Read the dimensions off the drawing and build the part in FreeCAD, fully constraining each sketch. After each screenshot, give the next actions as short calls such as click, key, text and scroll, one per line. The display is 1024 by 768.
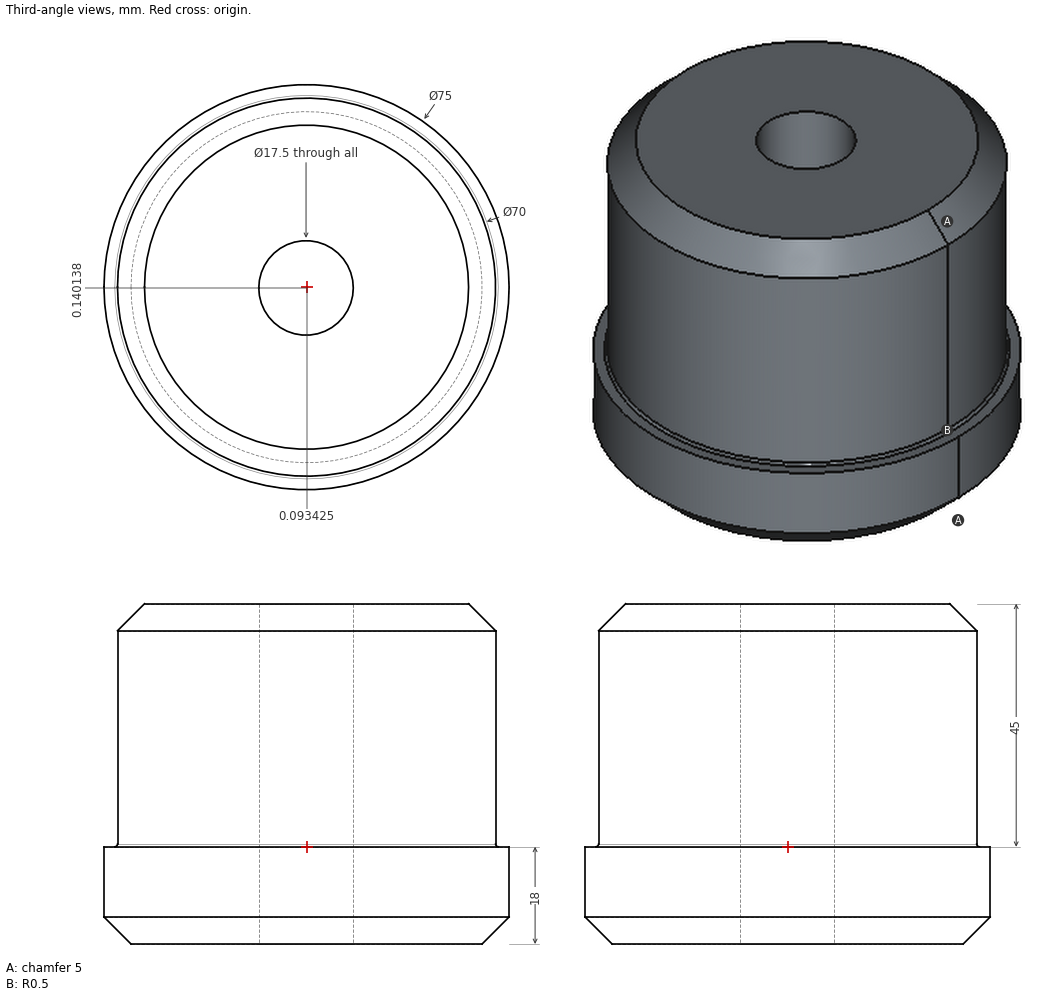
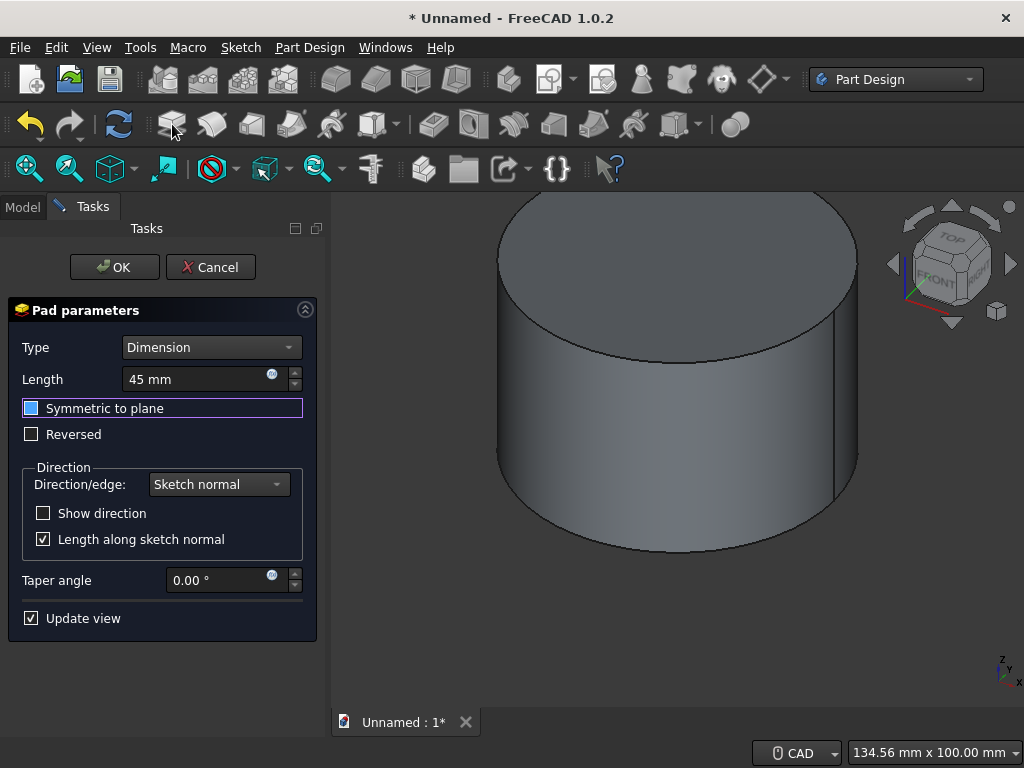
click(115, 267)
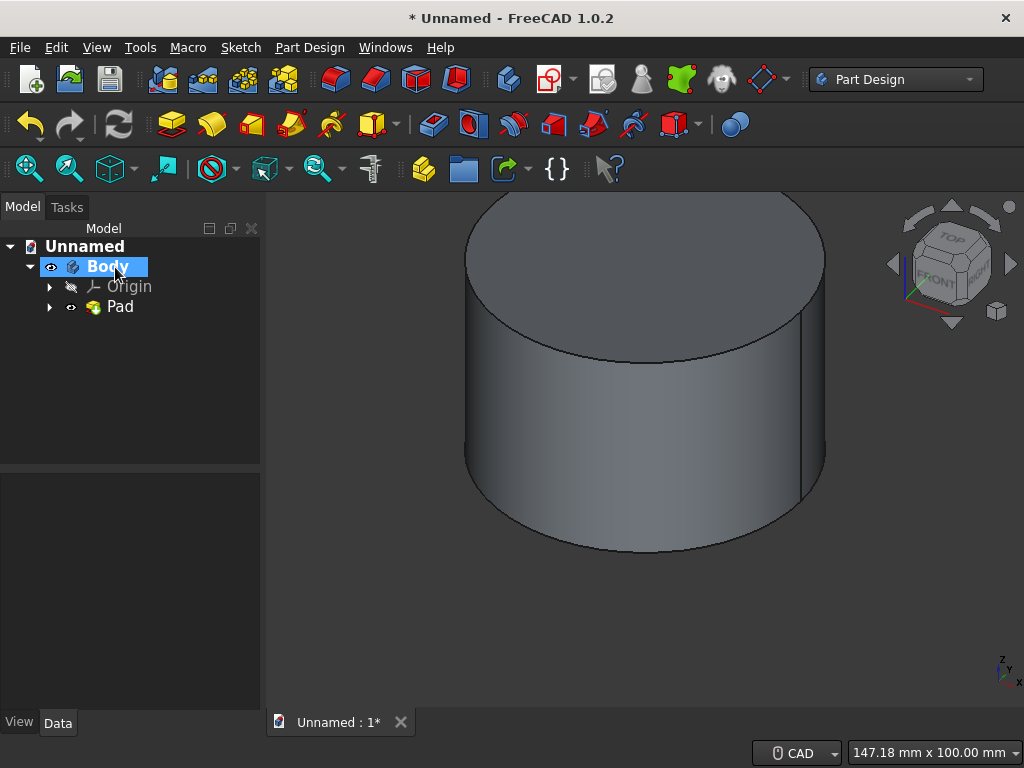
click(30, 170)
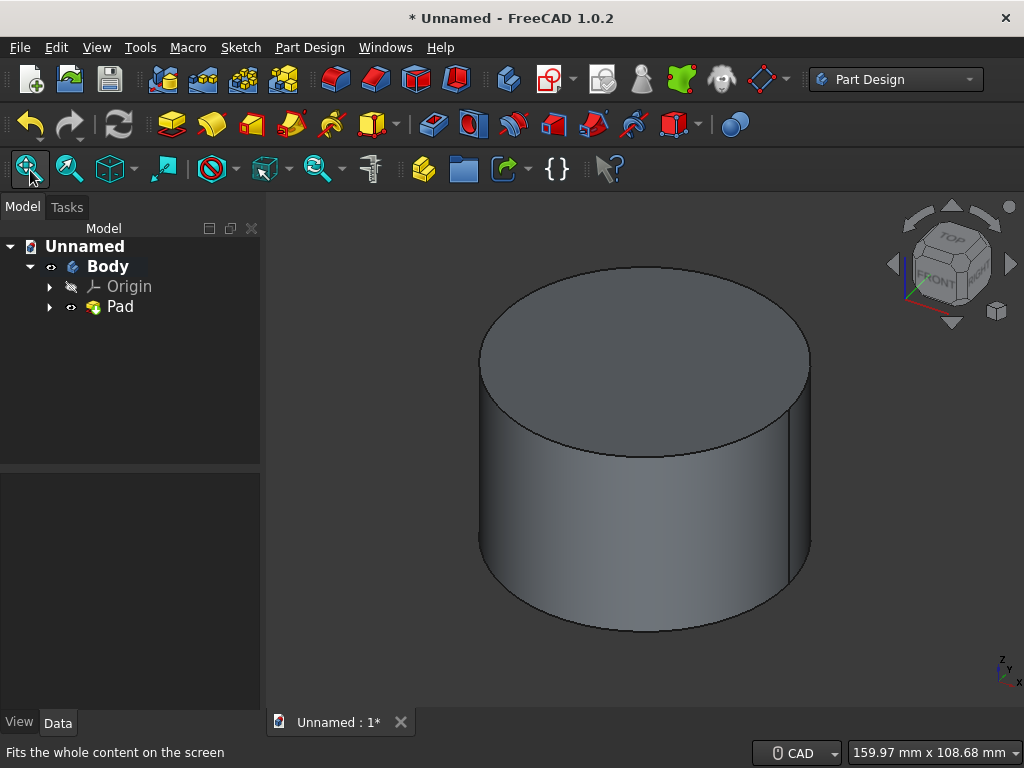
key(5)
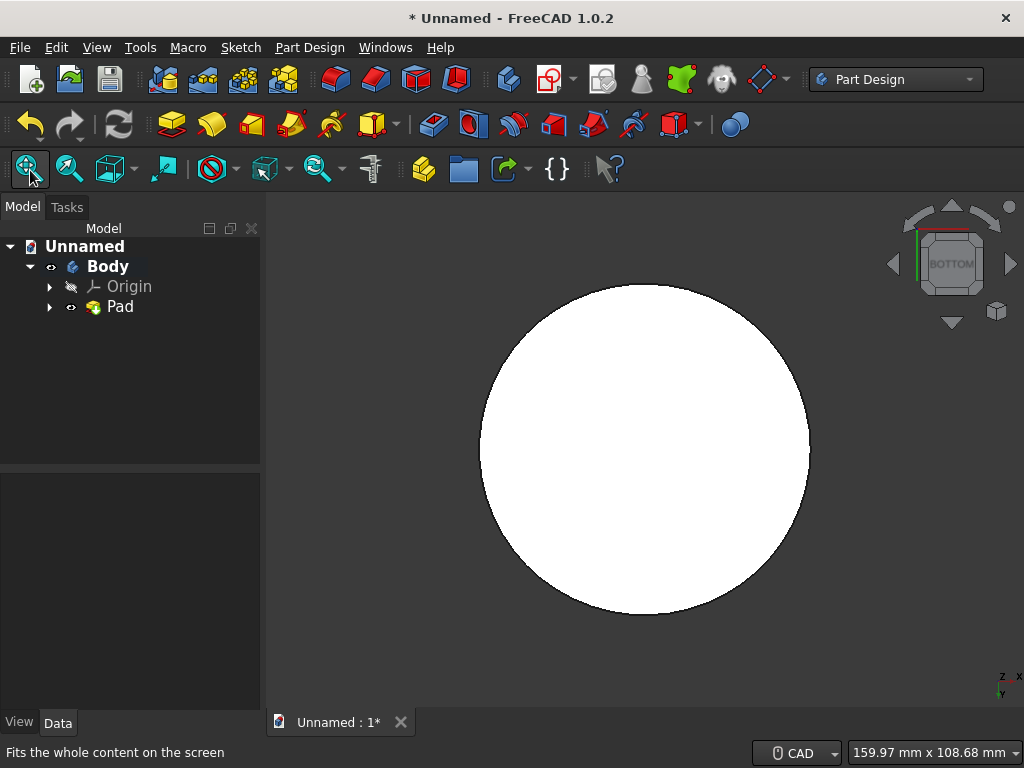
click(645, 448)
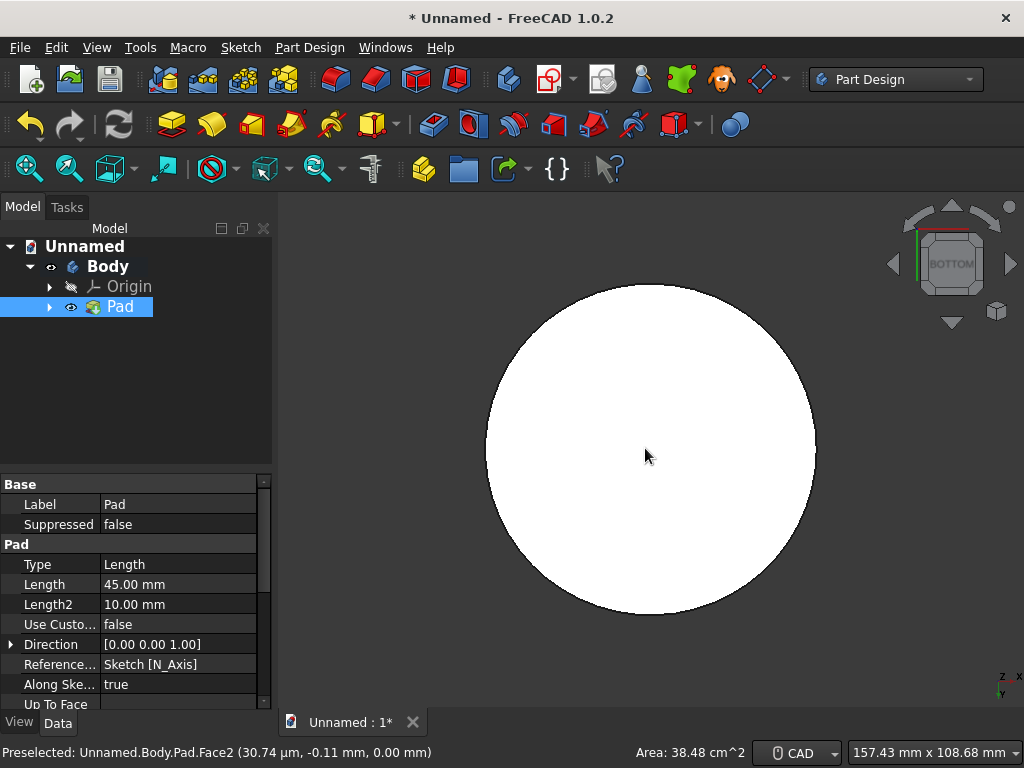
click(550, 80)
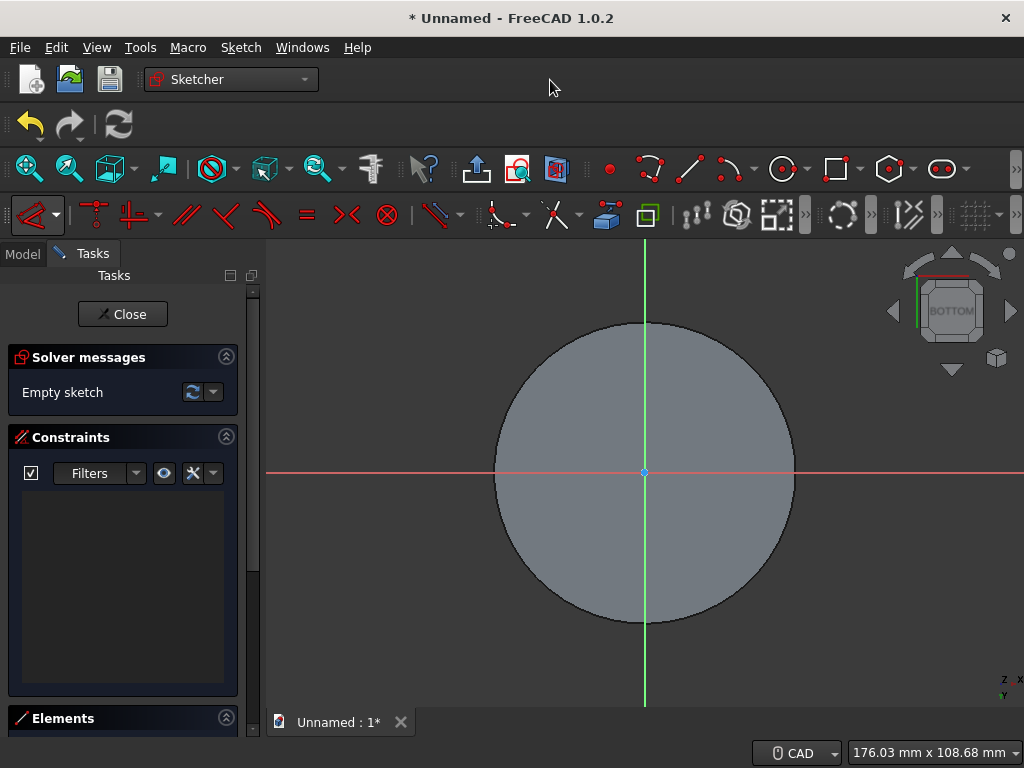
click(784, 170)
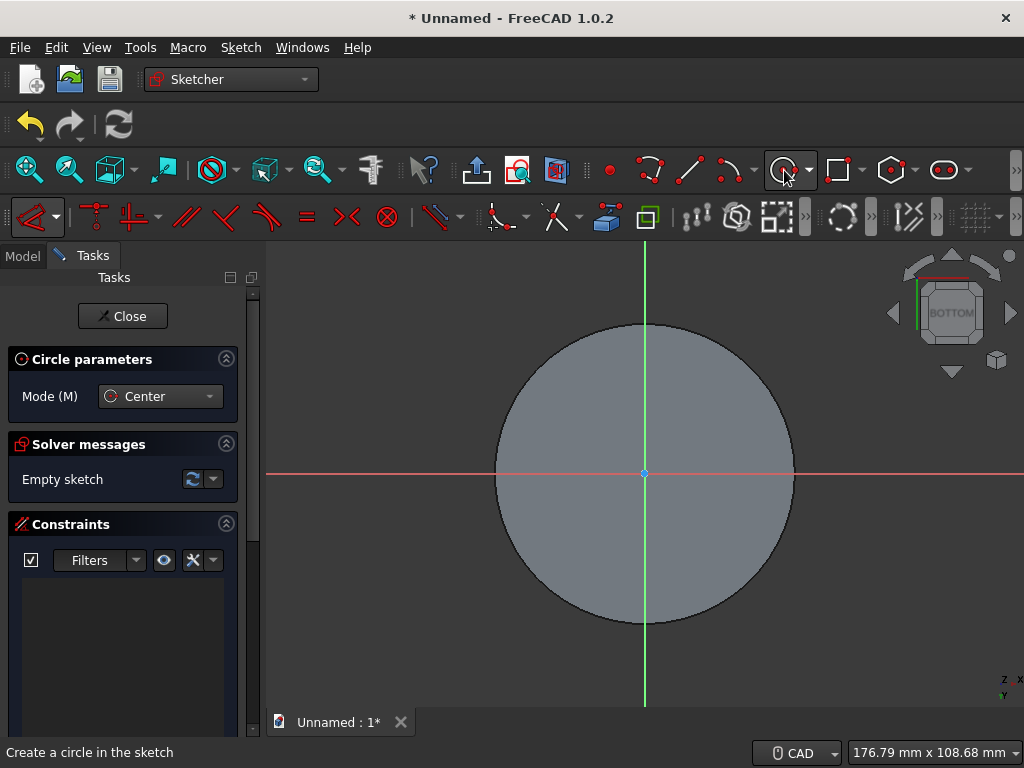
click(645, 474)
click(759, 360)
key(Escape)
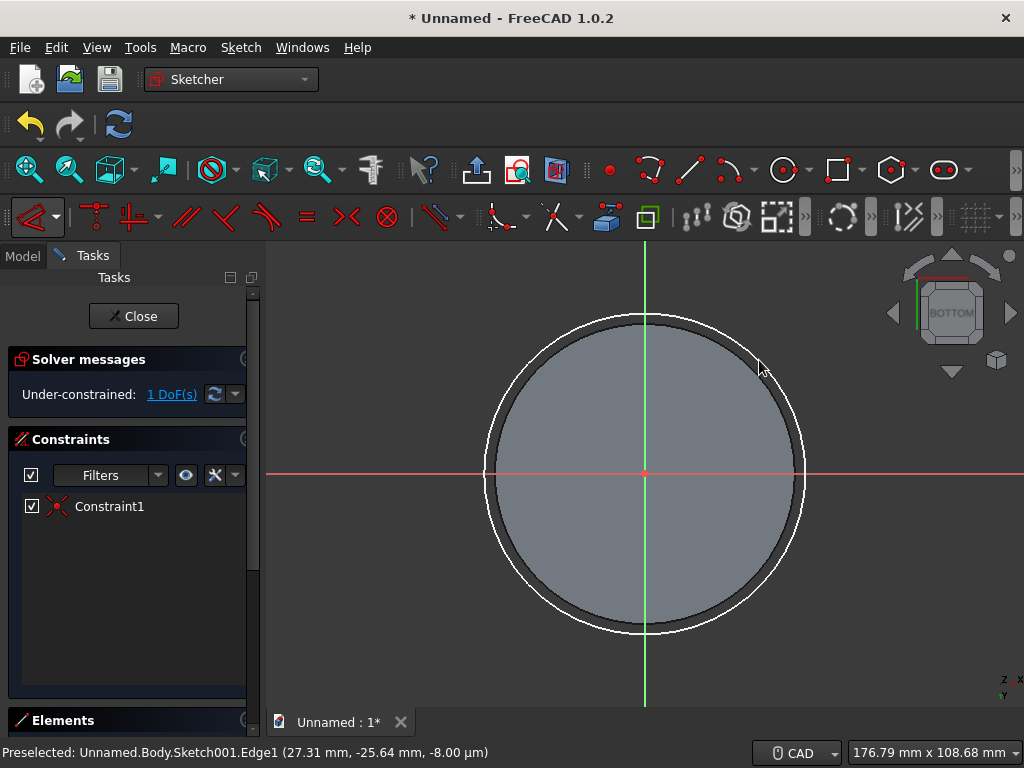
click(758, 360)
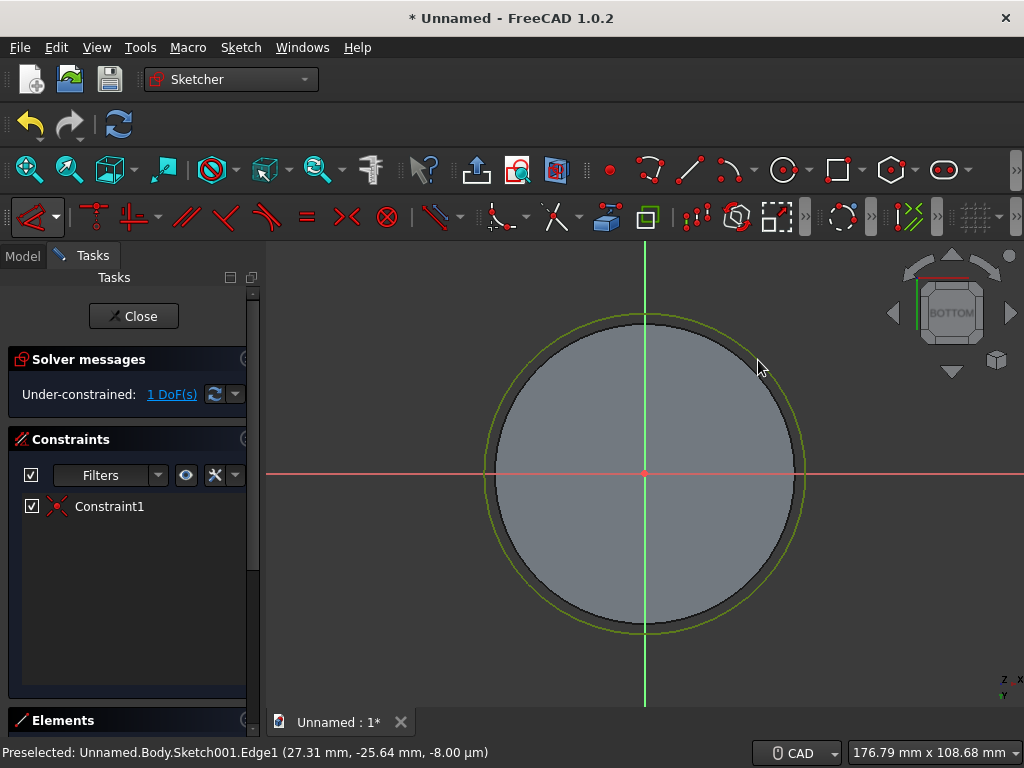
key(k)
key(o)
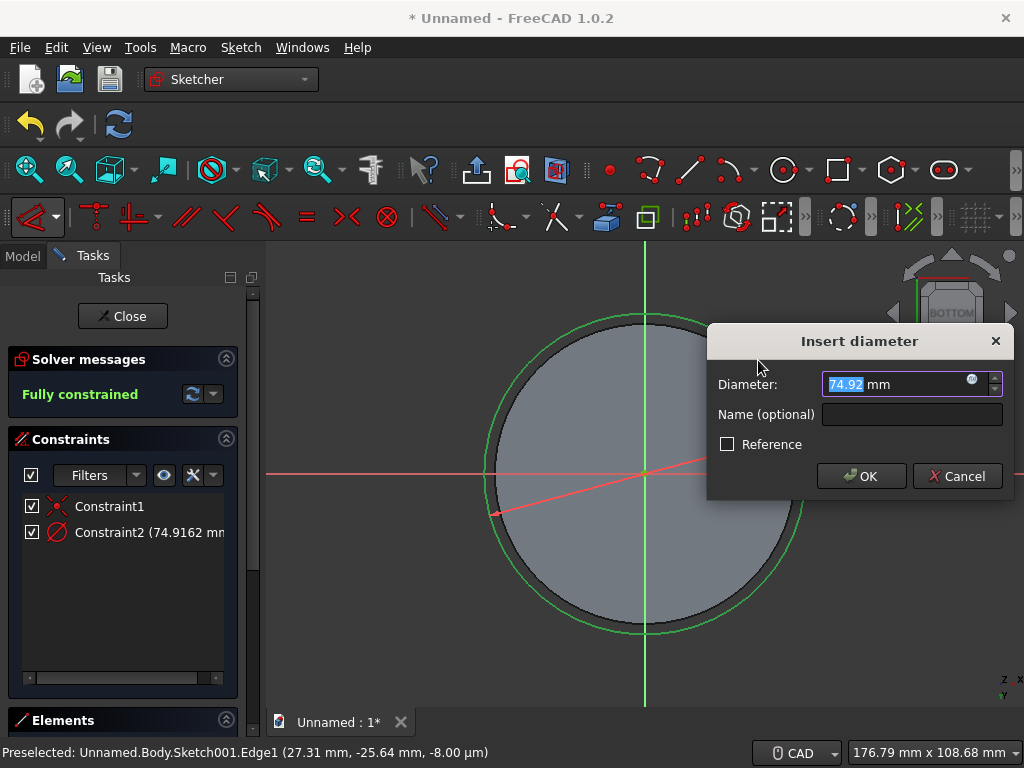
text(75)
key(Return)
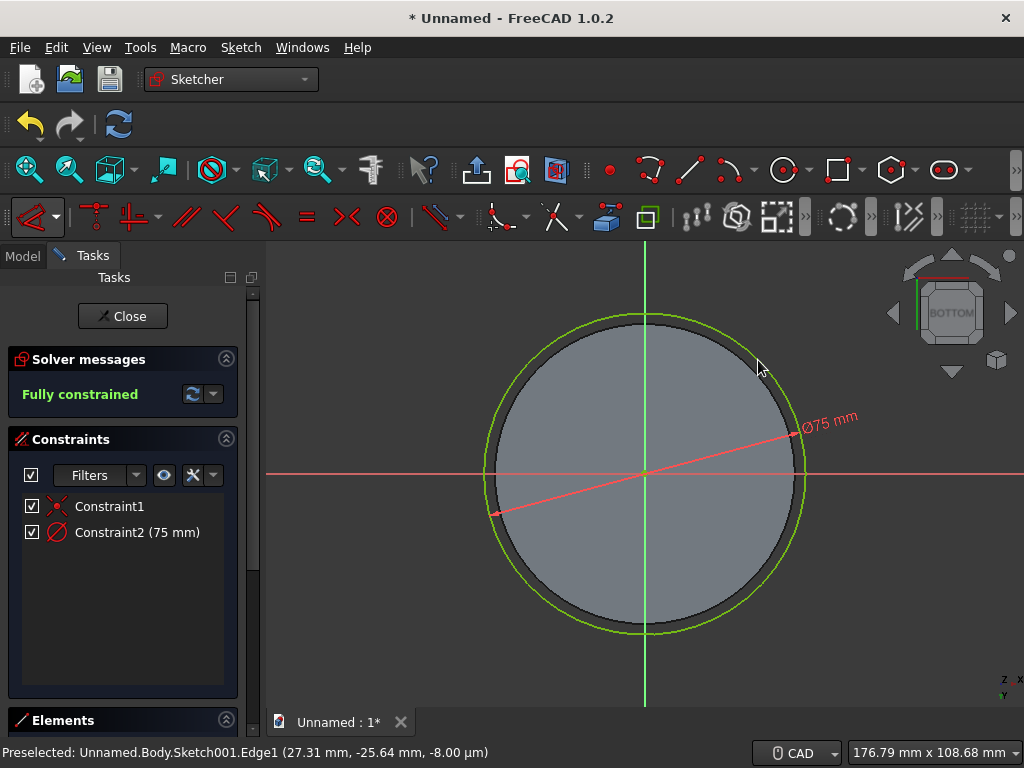
click(123, 316)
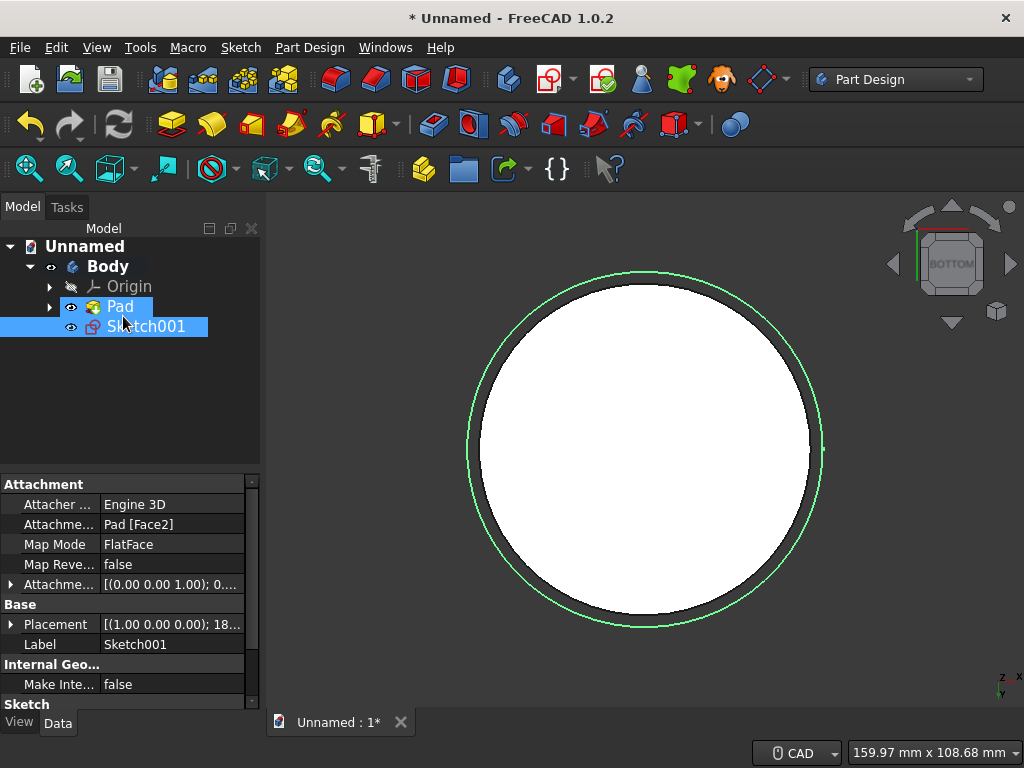
click(172, 124)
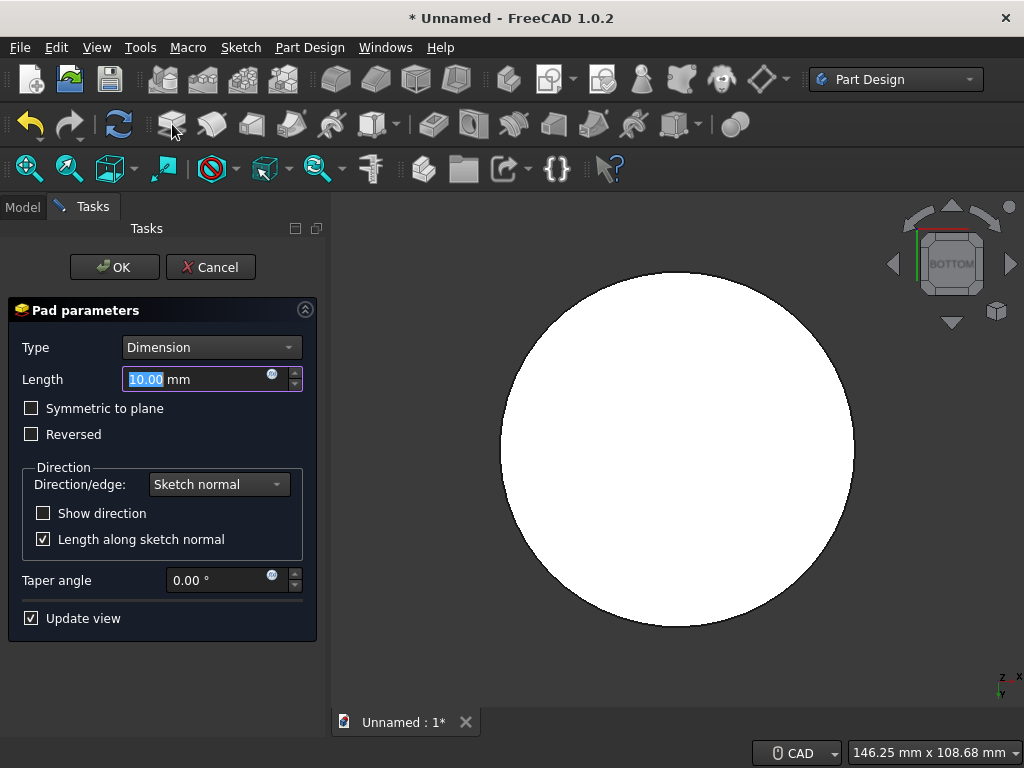
text(18)
key(Tab)